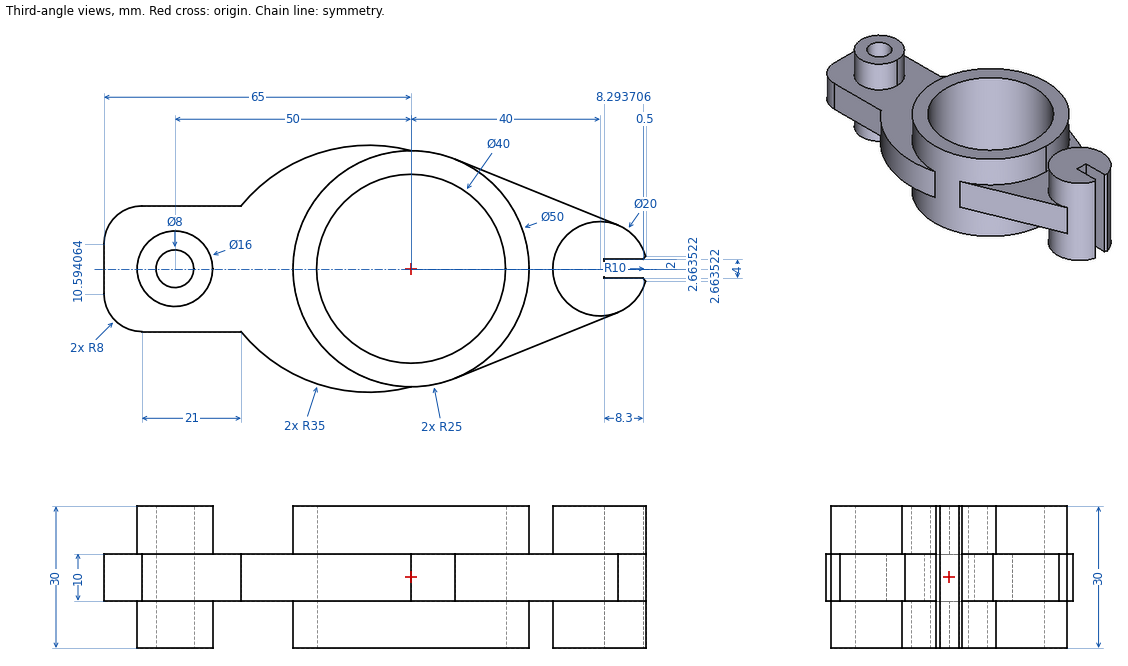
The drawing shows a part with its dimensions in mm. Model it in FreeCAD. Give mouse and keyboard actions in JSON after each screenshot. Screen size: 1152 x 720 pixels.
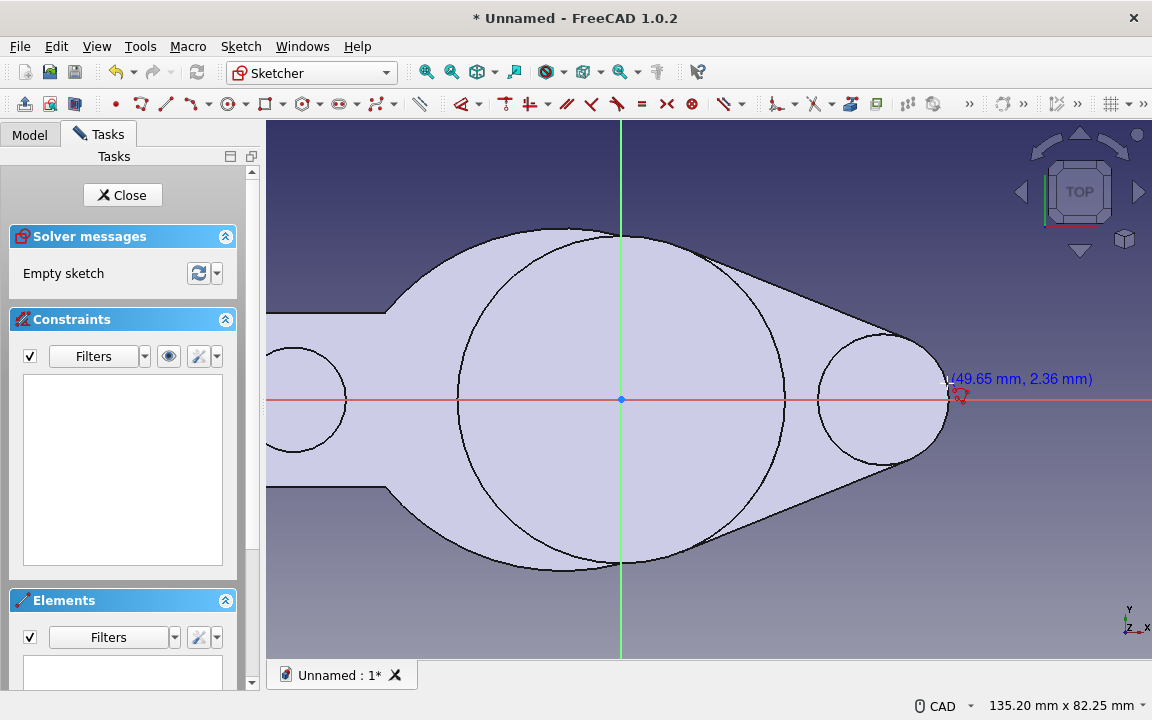
{"action": "left_click", "coordinate": [947, 382]}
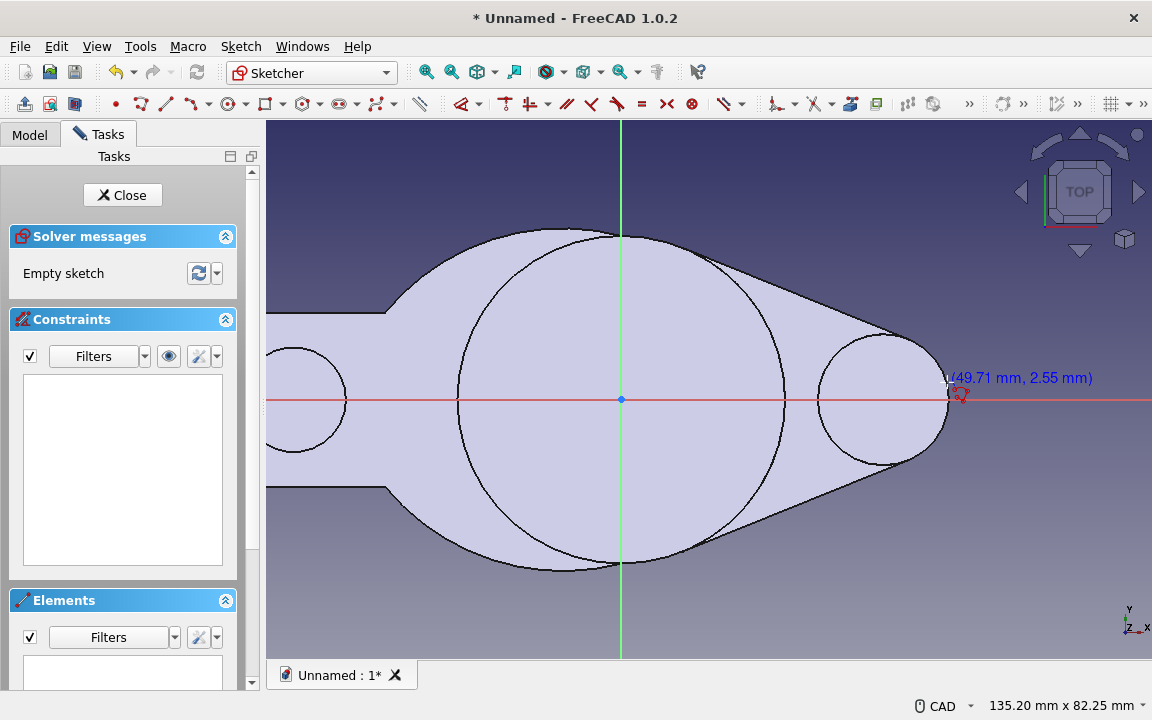
{"action": "scroll", "coordinate": [943, 387], "scroll_direction": "up", "scroll_amount": 6}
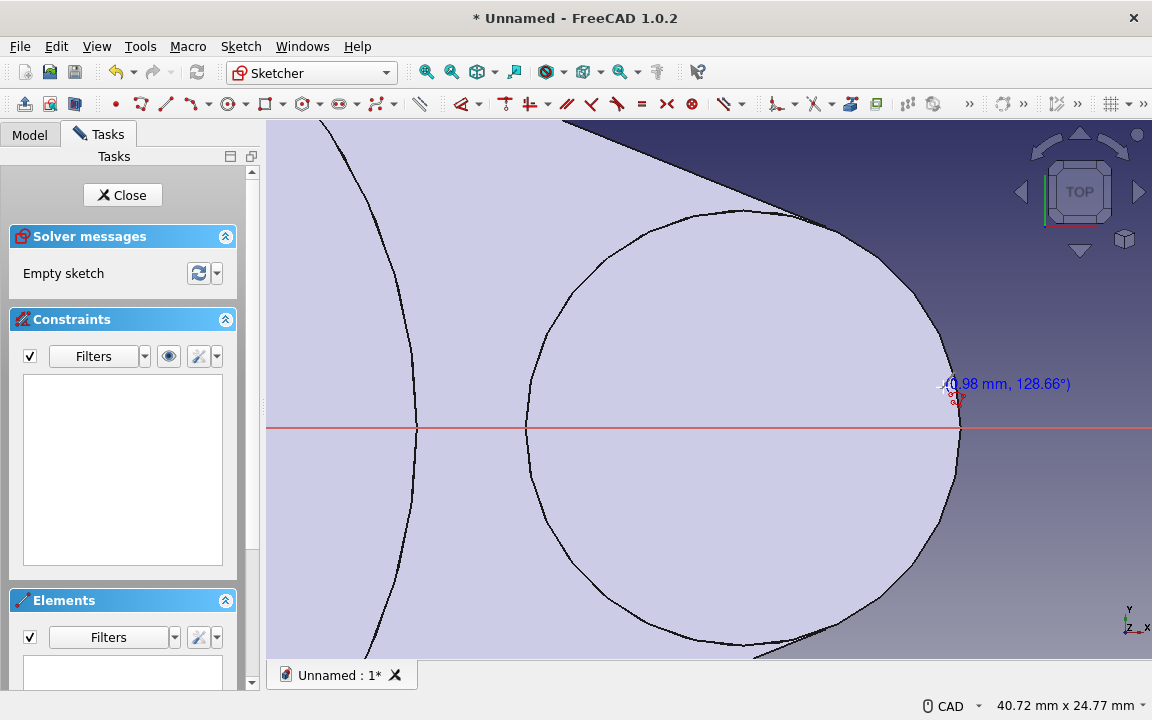
{"action": "left_click", "coordinate": [942, 385]}
{"action": "left_click", "coordinate": [762, 385]}
{"action": "left_click", "coordinate": [762, 472]}
{"action": "left_click", "coordinate": [942, 472]}
{"action": "left_click", "coordinate": [953, 486]}
{"action": "right_click", "coordinate": [953, 486]}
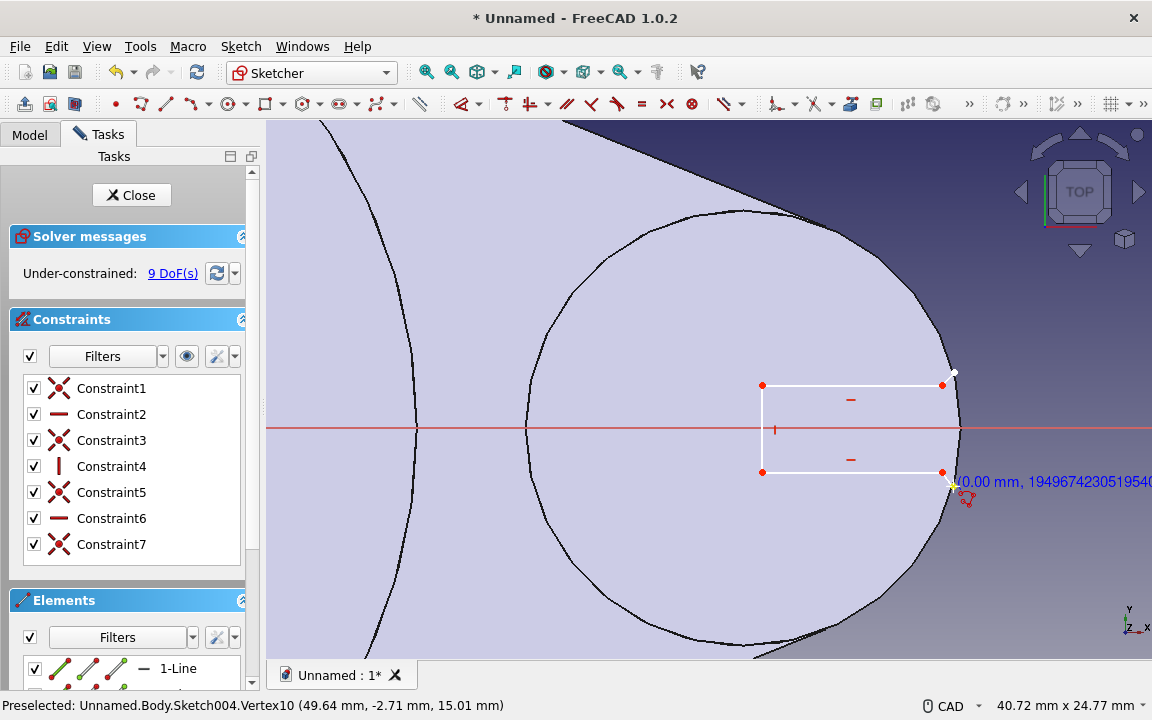
{"action": "left_click", "coordinate": [190, 104]}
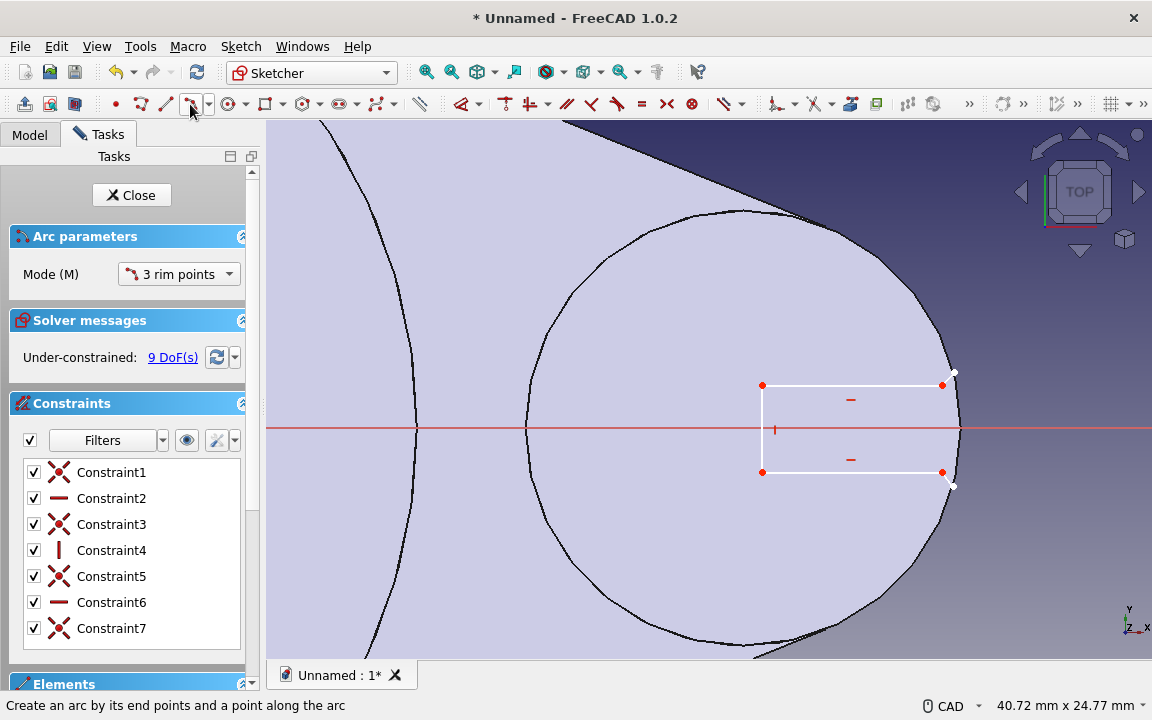
{"action": "scroll", "coordinate": [953, 486], "scroll_direction": "up", "scroll_amount": 3}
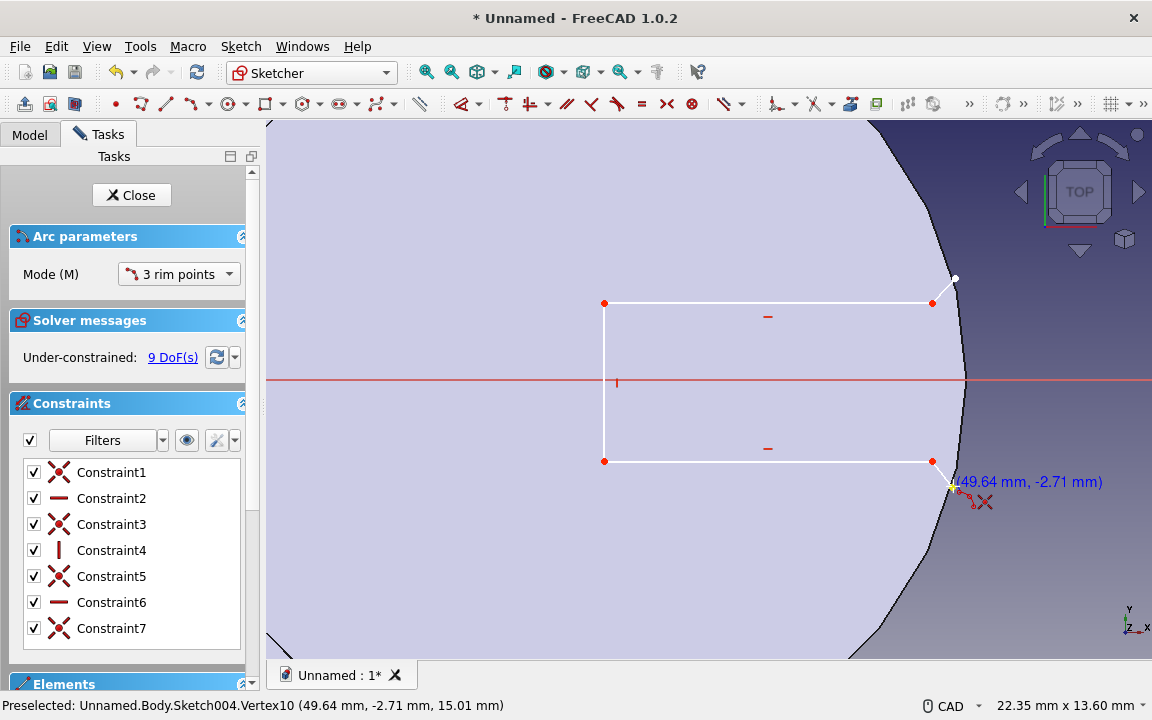
{"action": "left_click", "coordinate": [952, 487]}
{"action": "left_click", "coordinate": [955, 279]}
{"action": "left_click", "coordinate": [966, 401]}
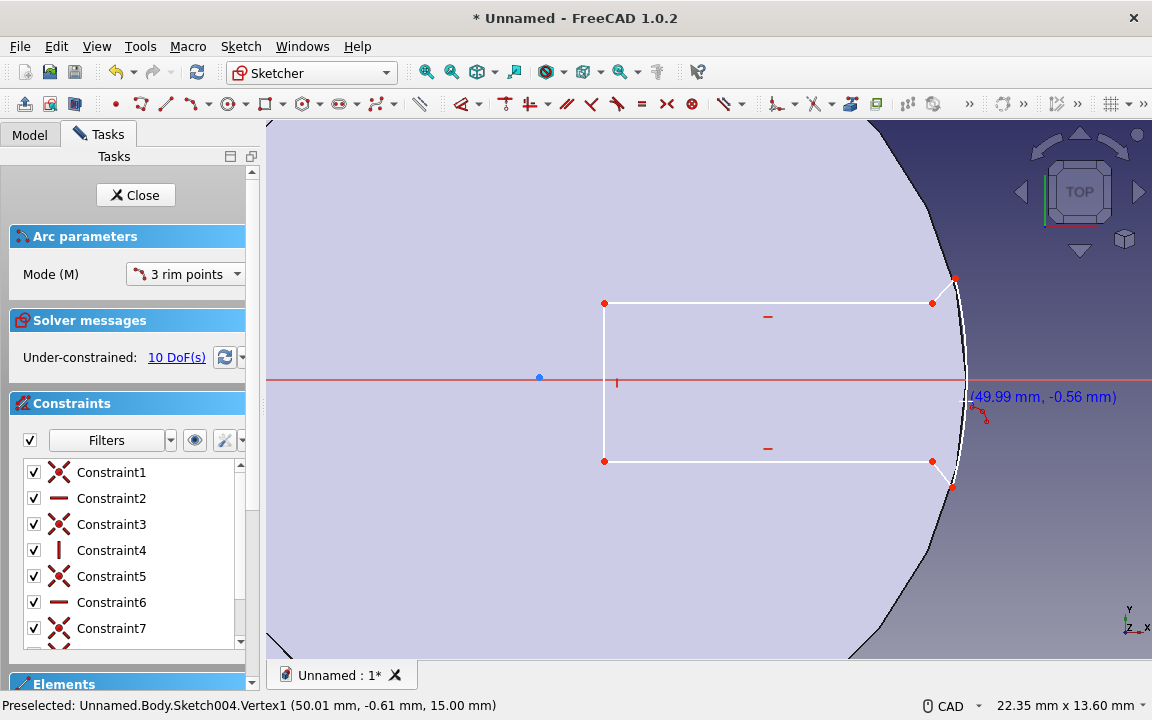
{"action": "left_click", "coordinate": [228, 104]}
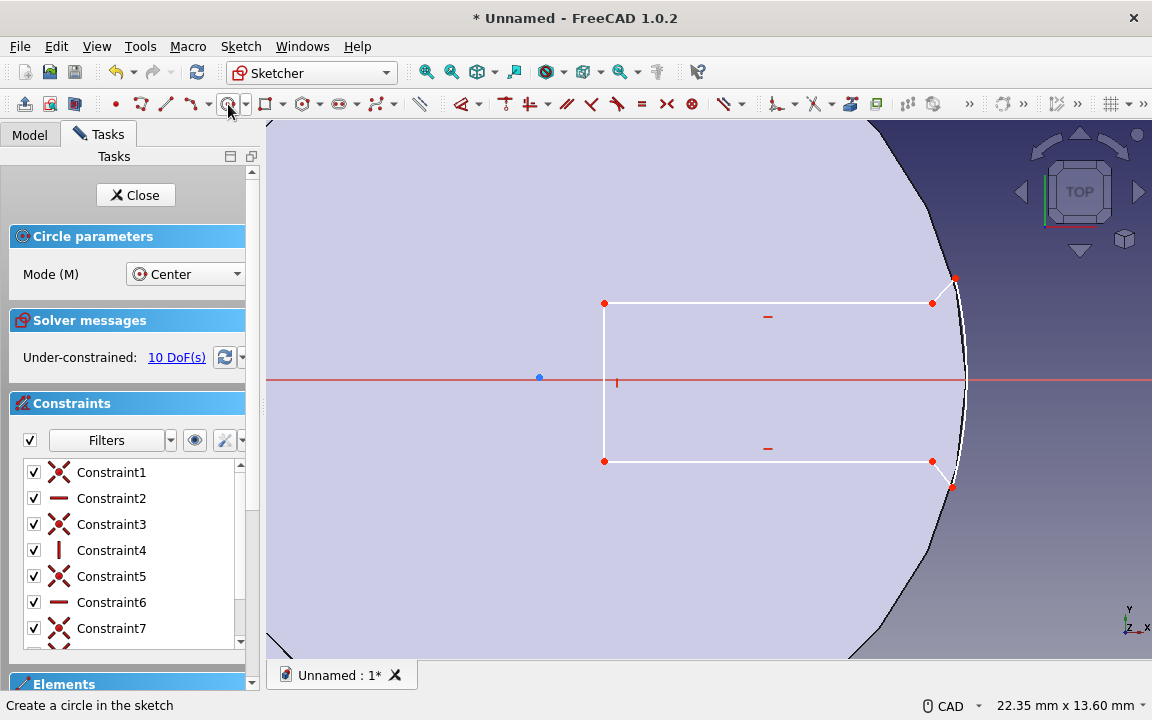
{"action": "scroll", "coordinate": [857, 391], "scroll_direction": "down", "scroll_amount": 11}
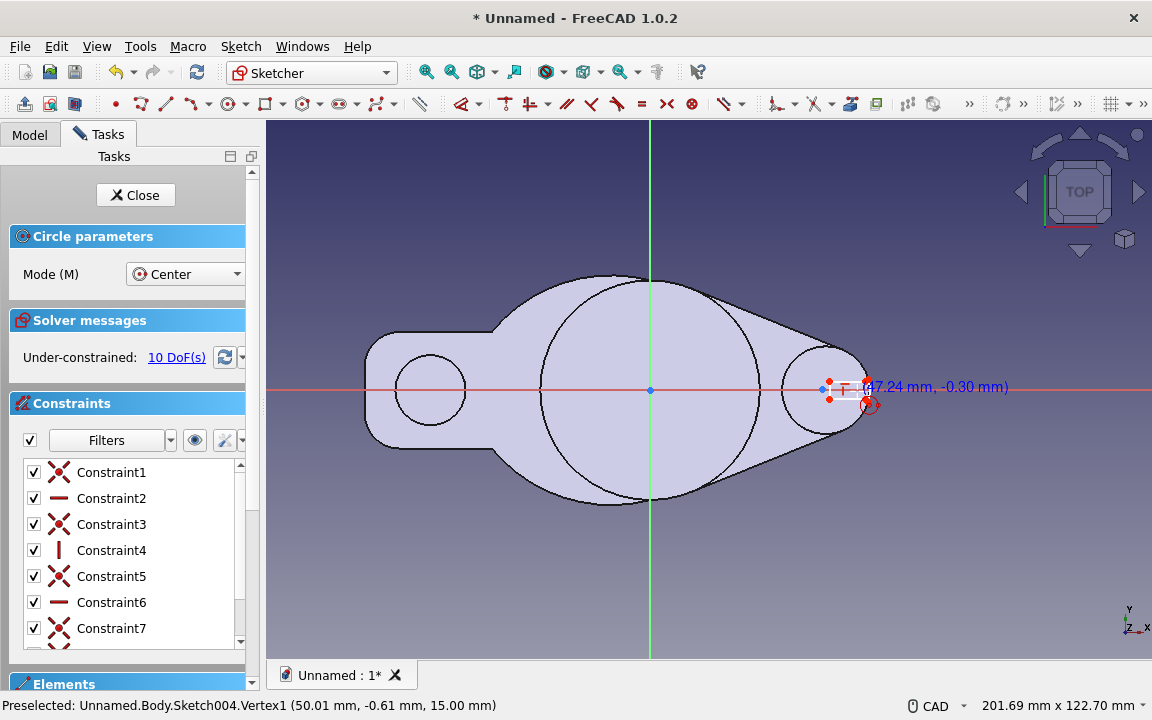
{"action": "left_click", "coordinate": [650, 390]}
{"action": "left_click", "coordinate": [712, 328]}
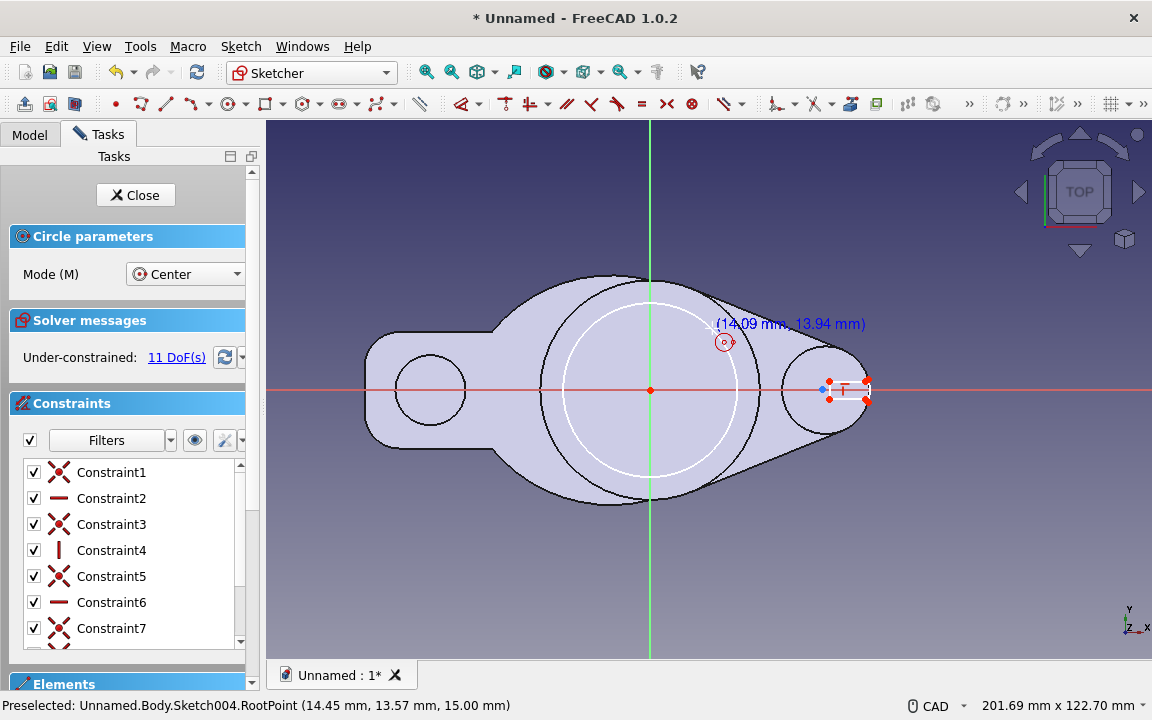
{"action": "scroll", "coordinate": [430, 390], "scroll_direction": "up", "scroll_amount": 2}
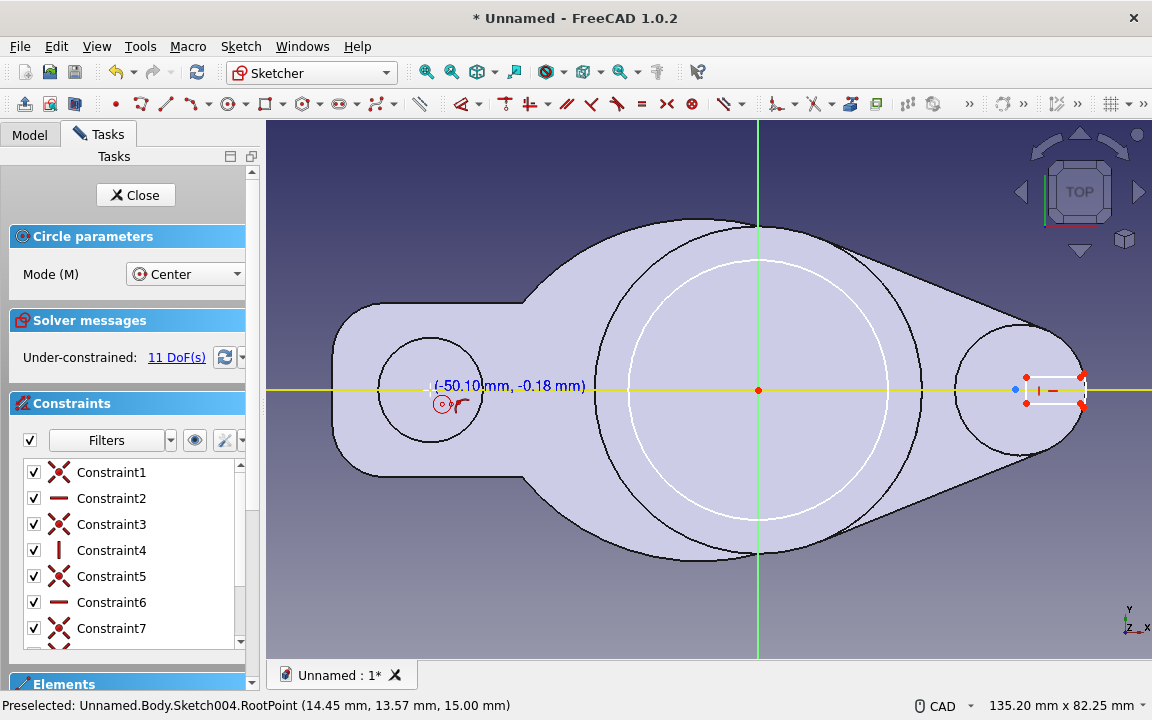
{"action": "left_click", "coordinate": [431, 390]}
{"action": "left_click", "coordinate": [449, 372]}
{"action": "key", "text": "Escape"}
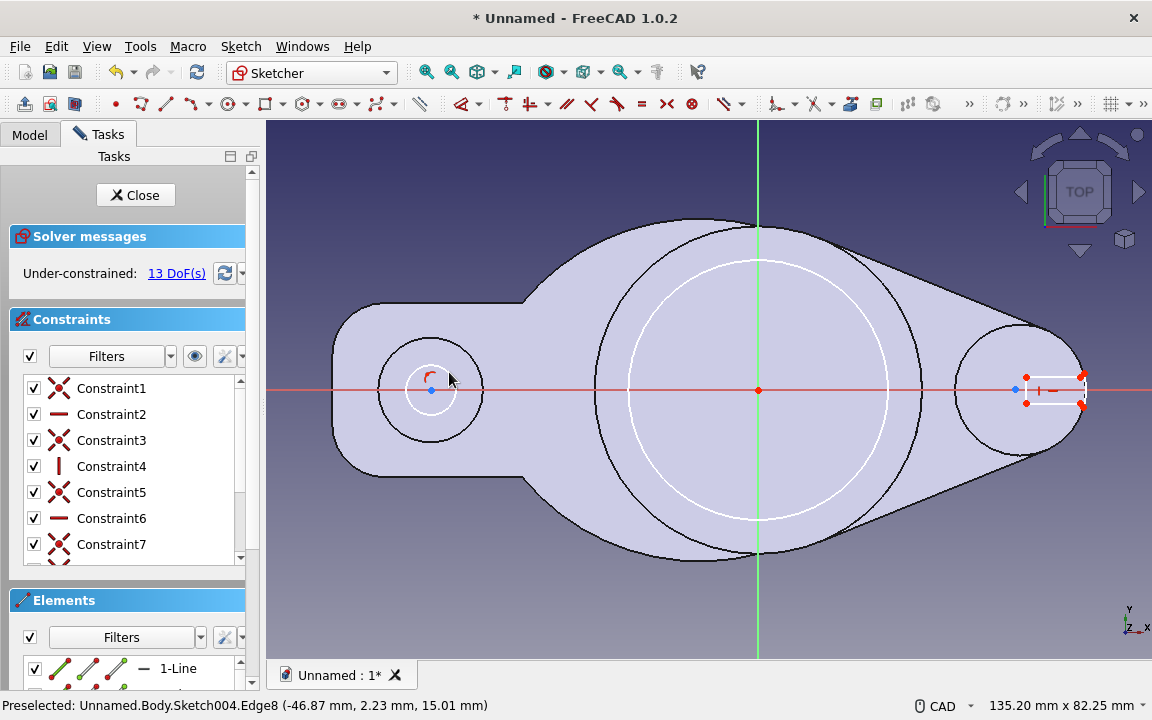
{"action": "scroll", "coordinate": [428, 388], "scroll_direction": "down", "scroll_amount": 2}